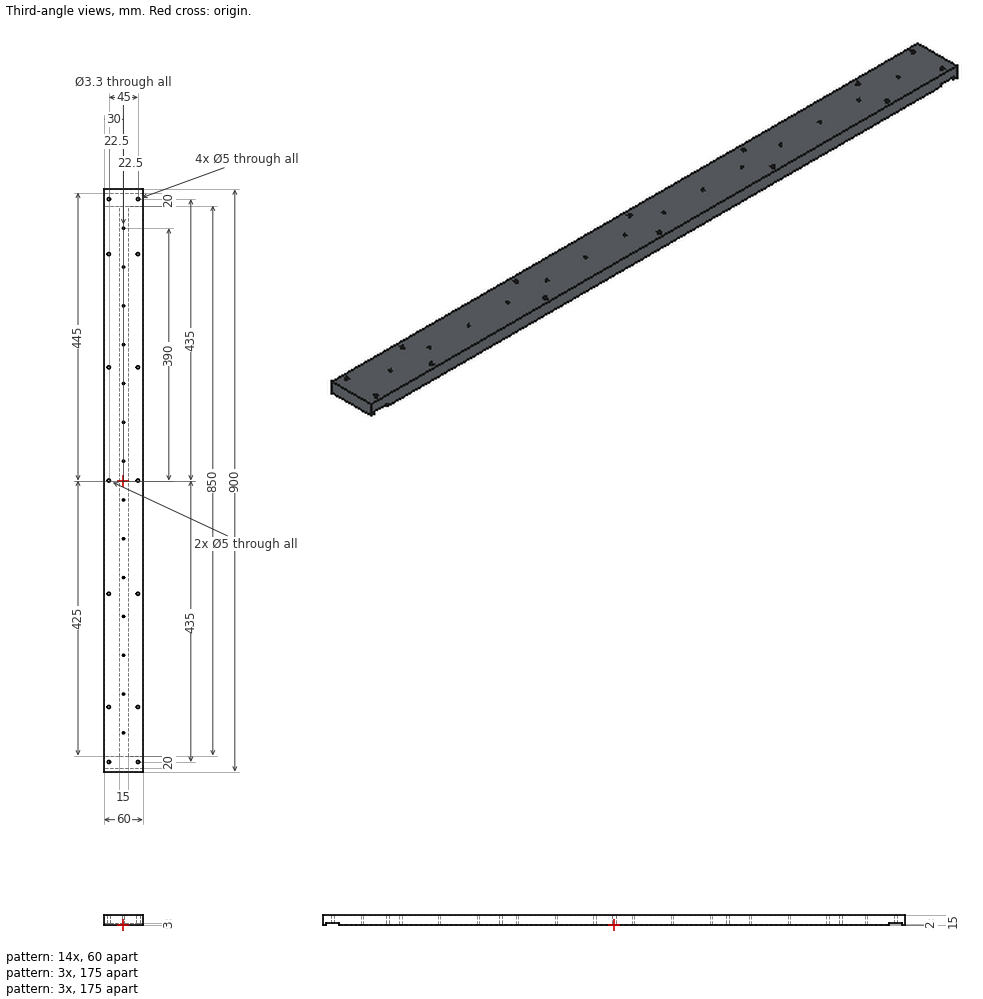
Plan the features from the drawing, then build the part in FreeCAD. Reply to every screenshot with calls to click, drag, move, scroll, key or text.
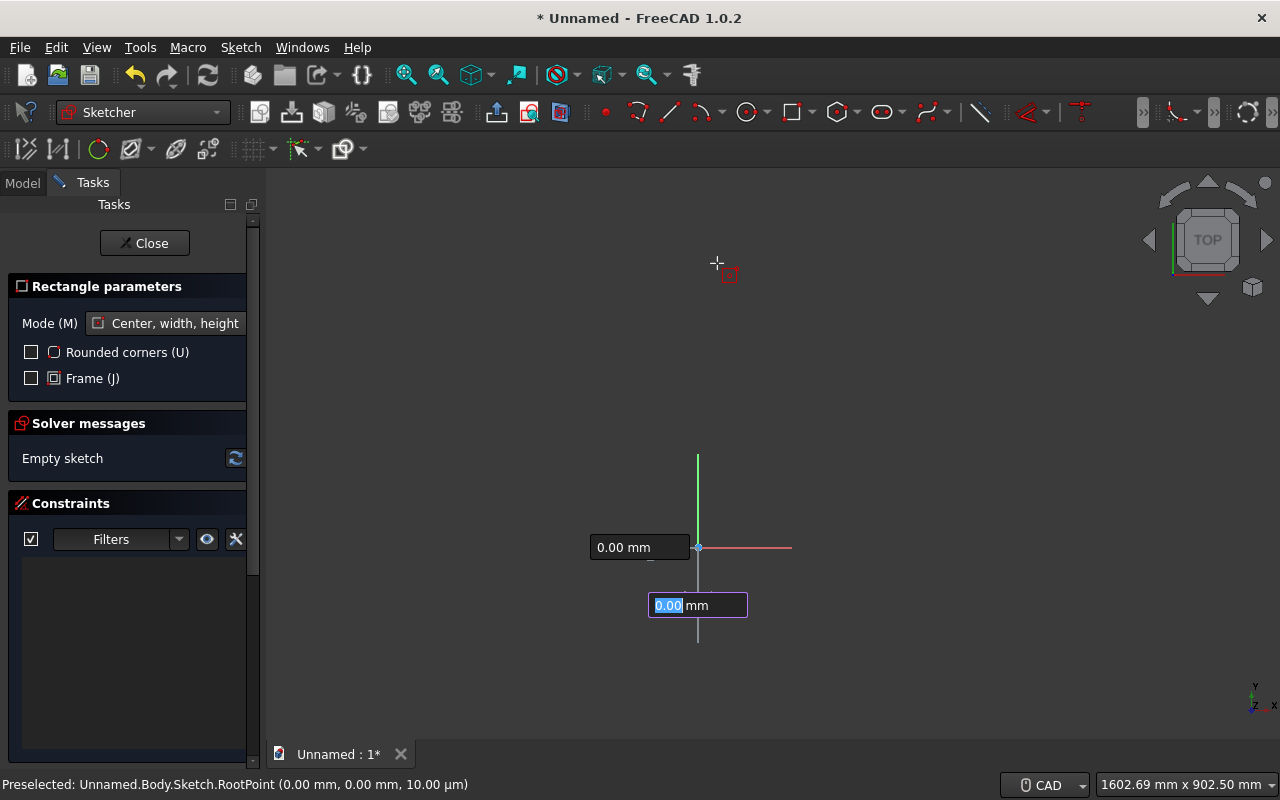
click(717, 263)
key(Escape)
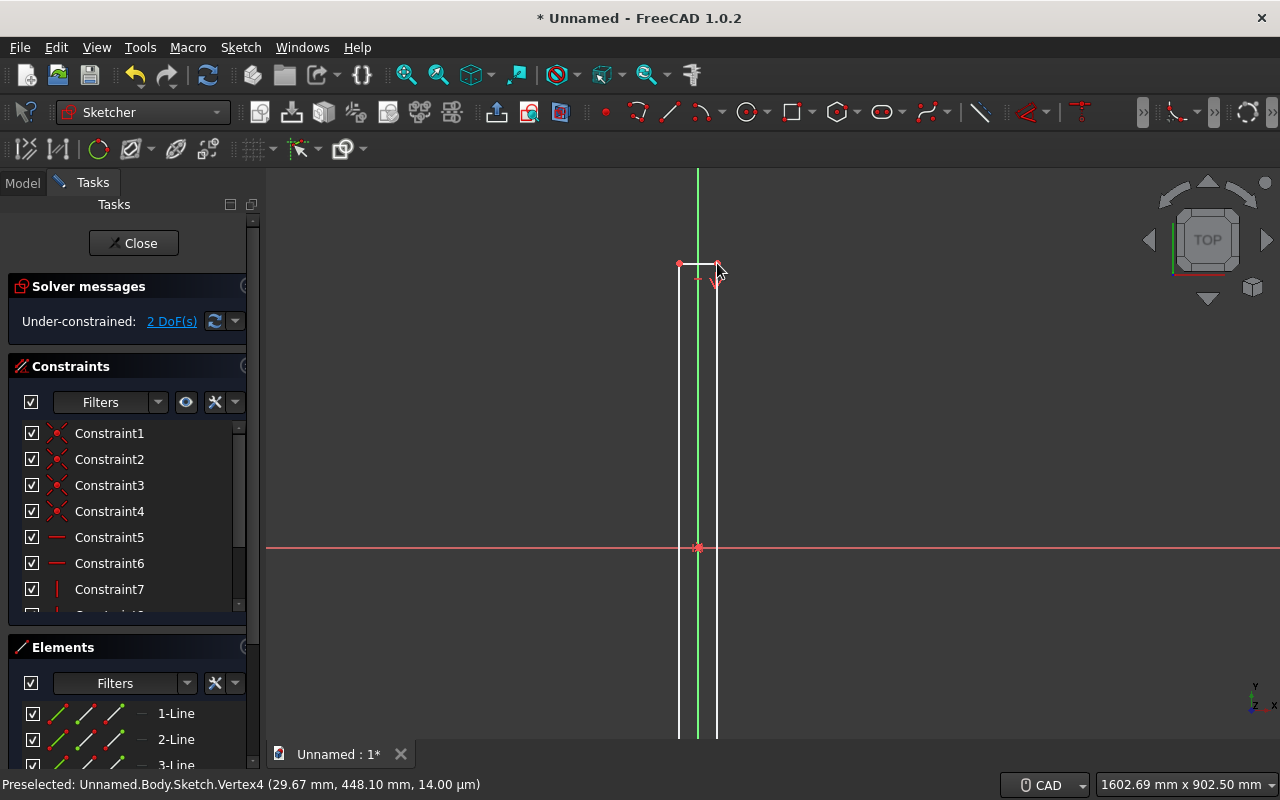
key(d)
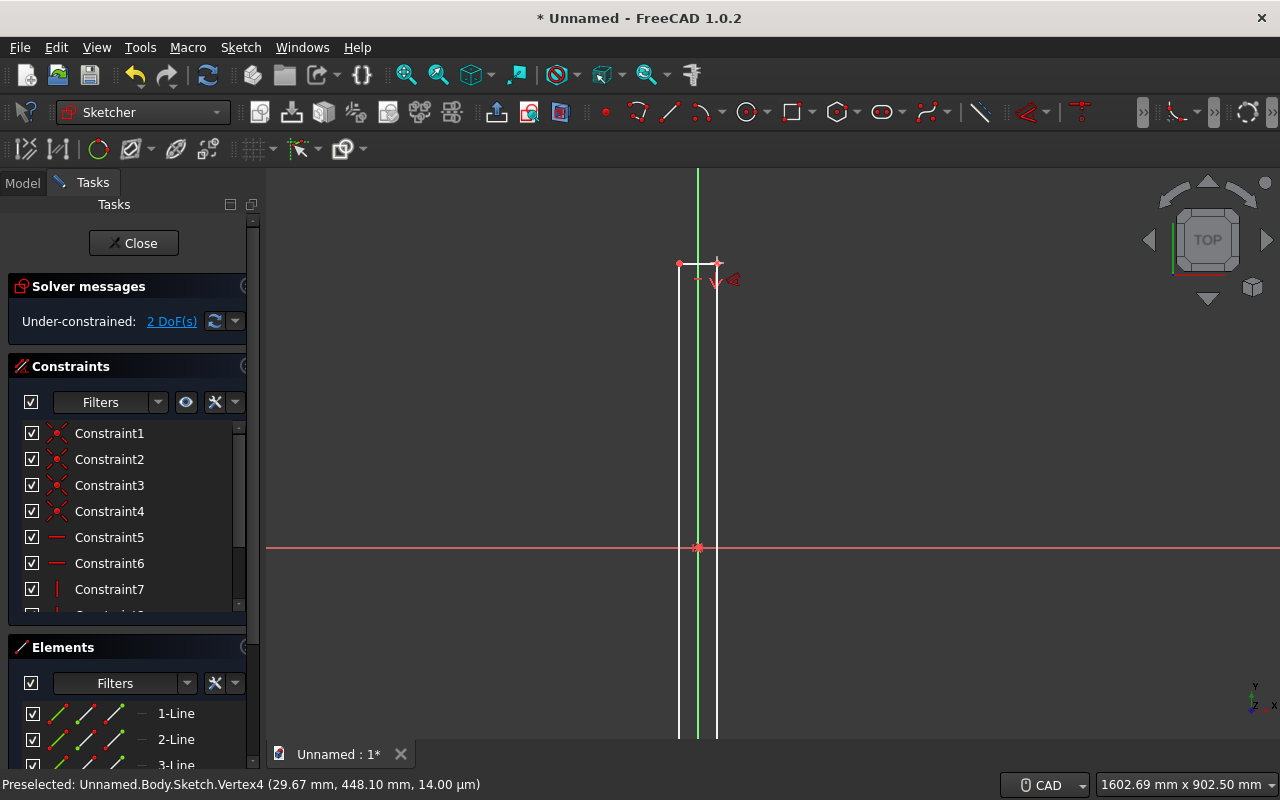
scroll(717, 262, down, 2)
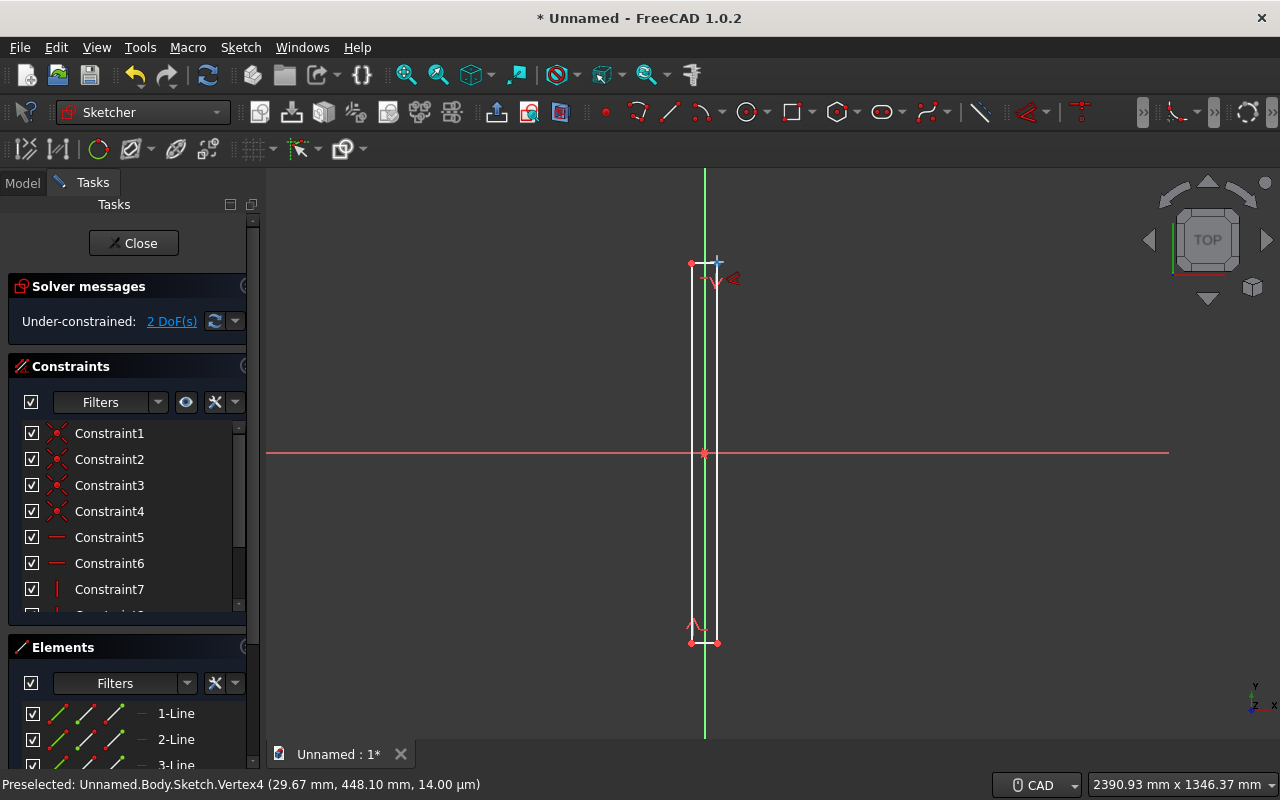
scroll(702, 643, up, 3)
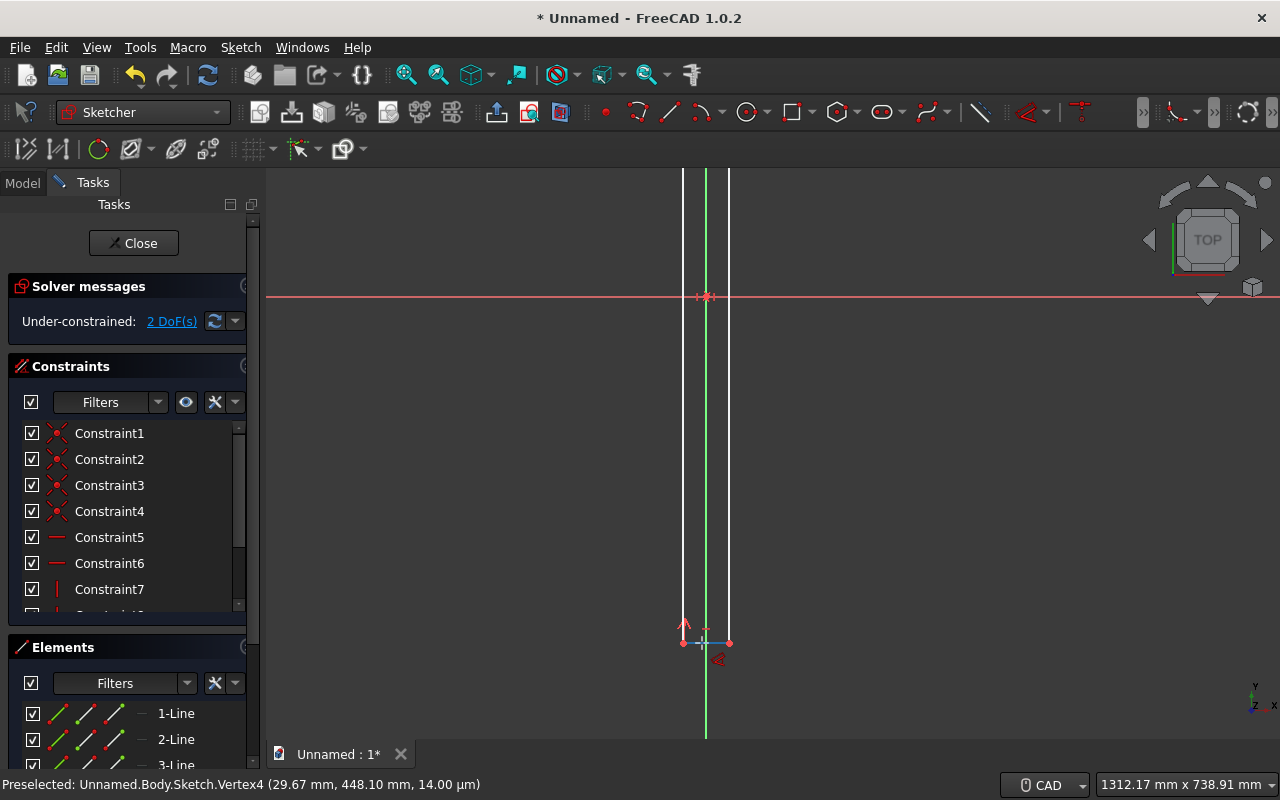
click(702, 643)
click(690, 677)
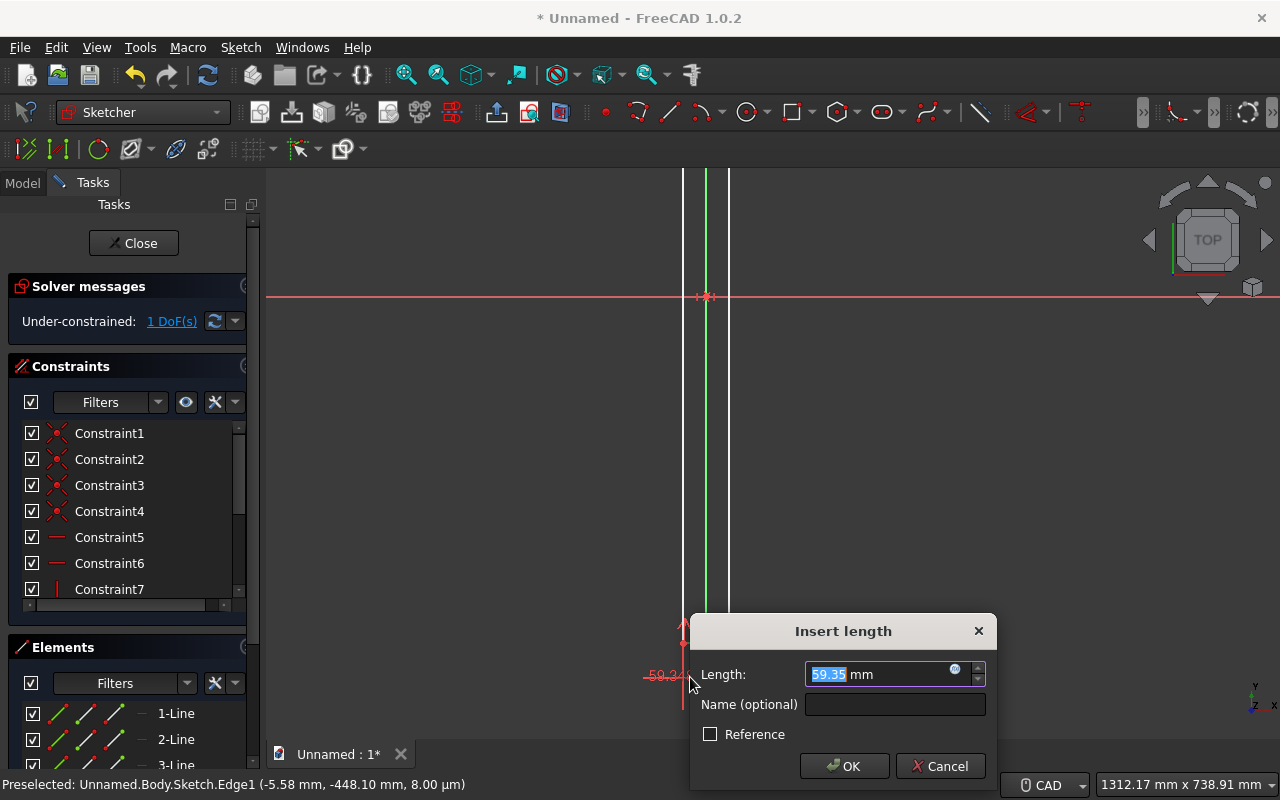
text(60)
key(Return)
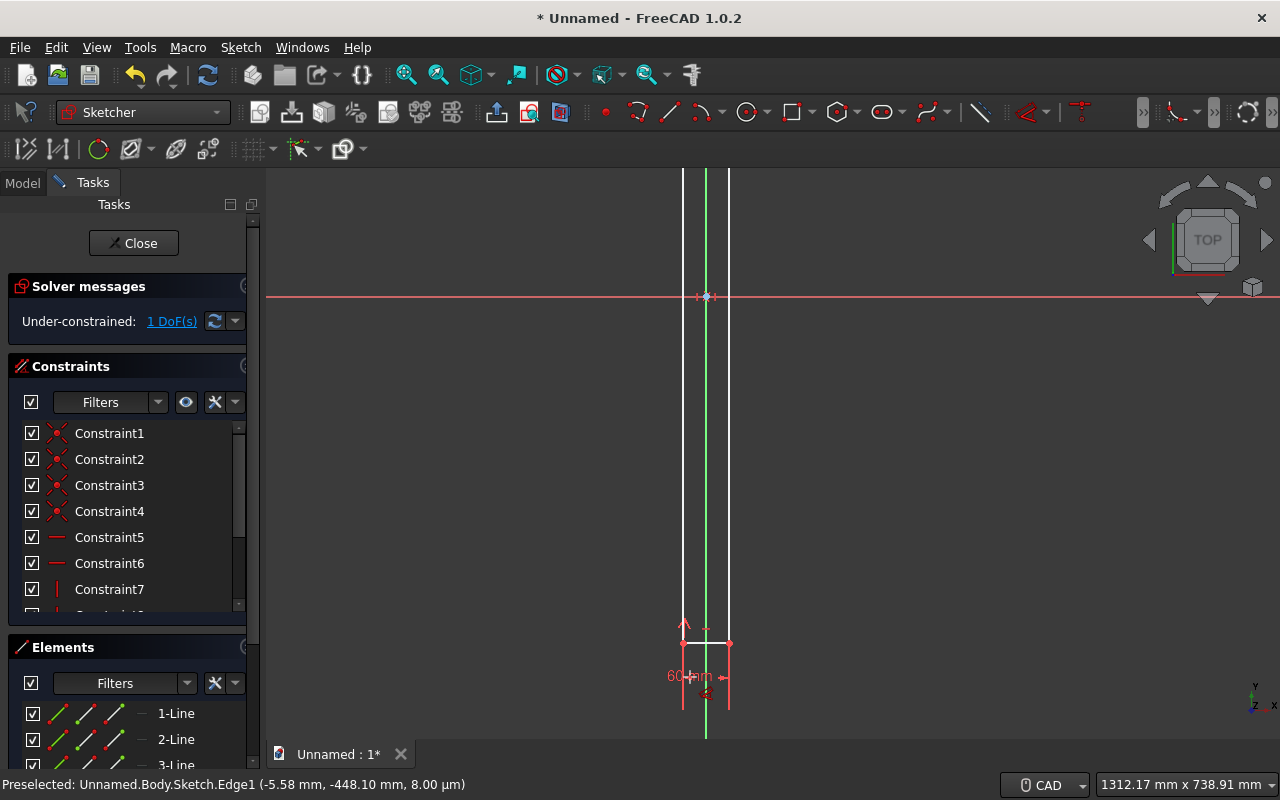
click(729, 435)
click(763, 420)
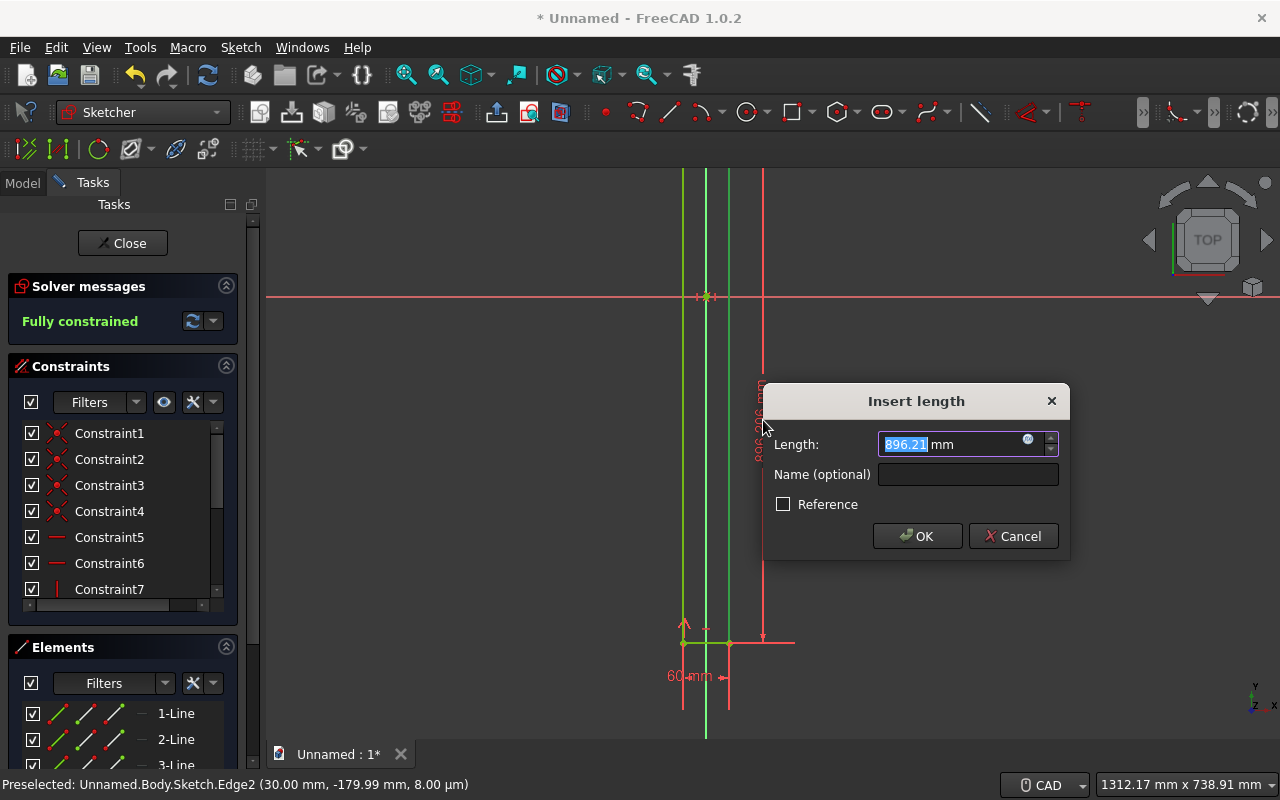
text(900)
key(Return)
key(Escape)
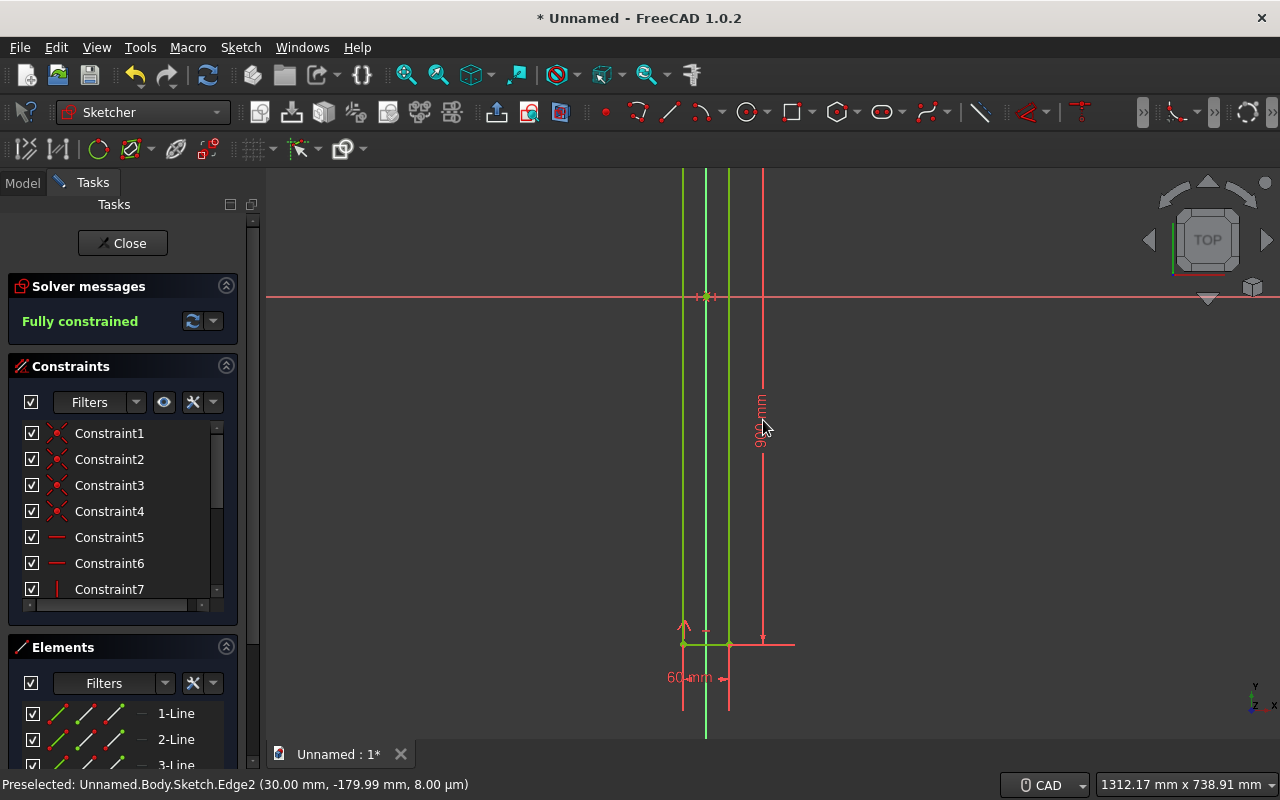
click(123, 243)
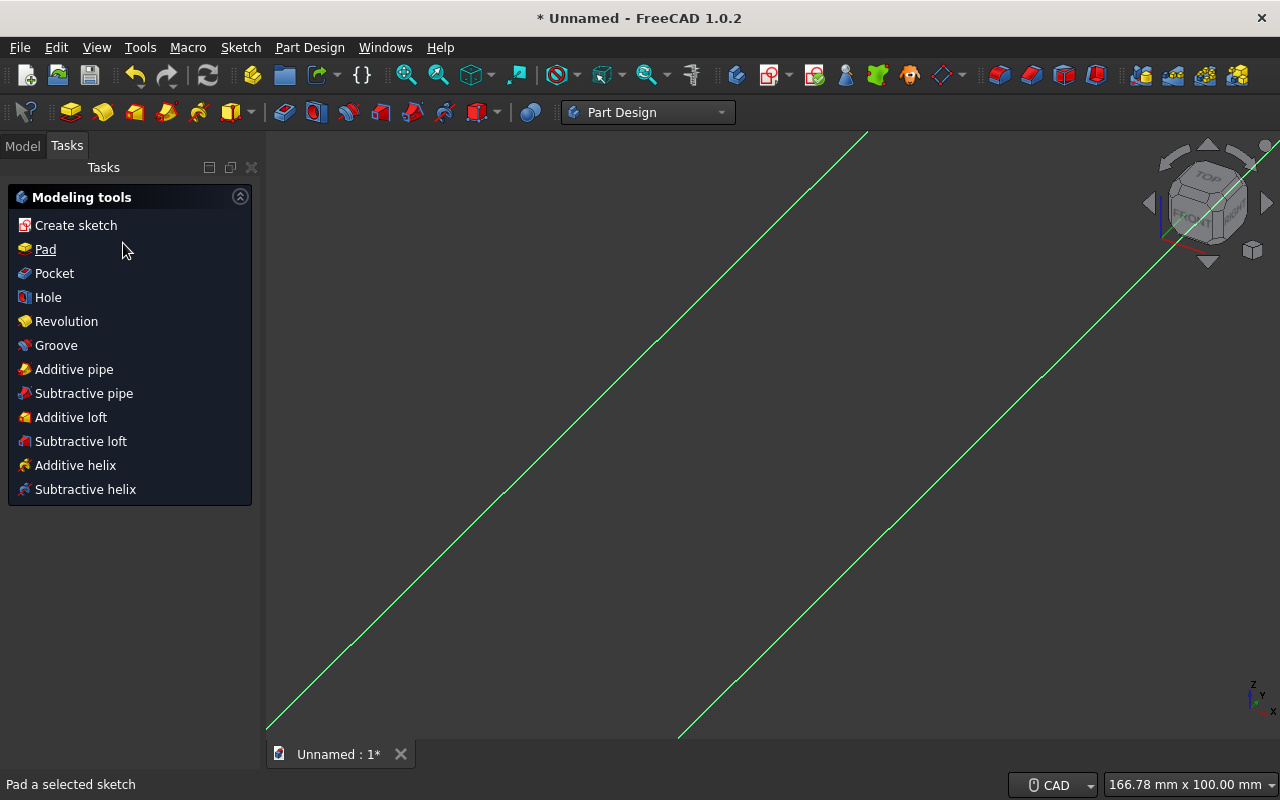
click(72, 112)